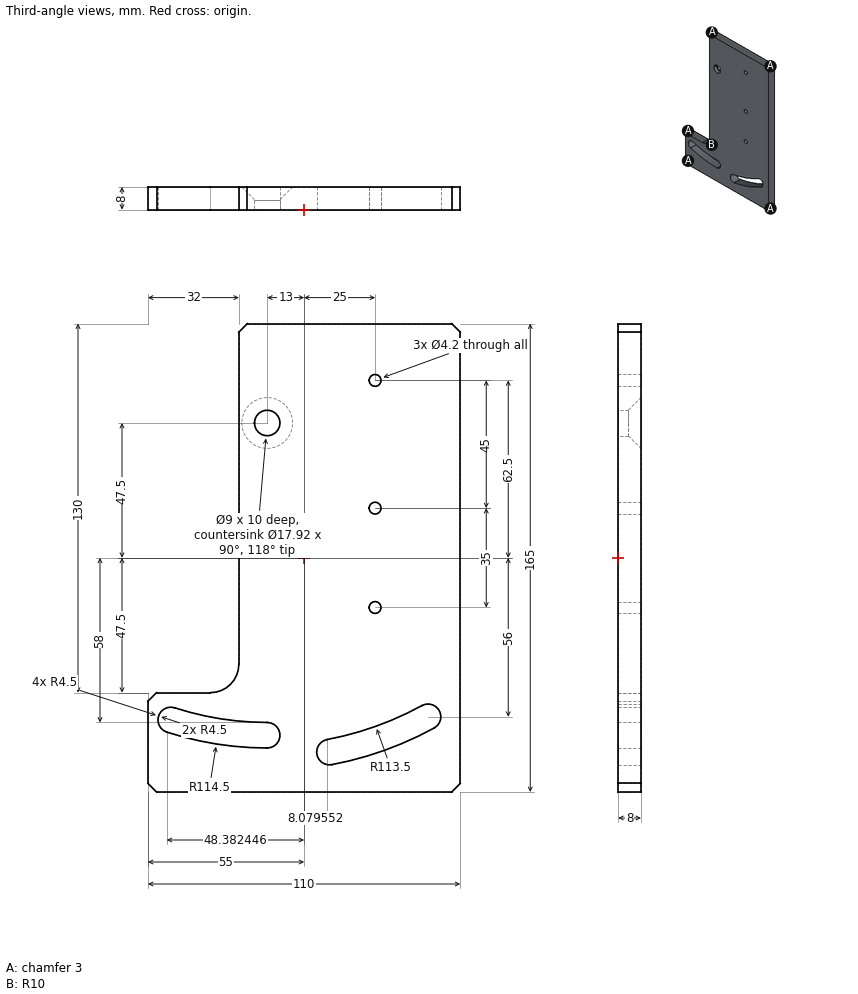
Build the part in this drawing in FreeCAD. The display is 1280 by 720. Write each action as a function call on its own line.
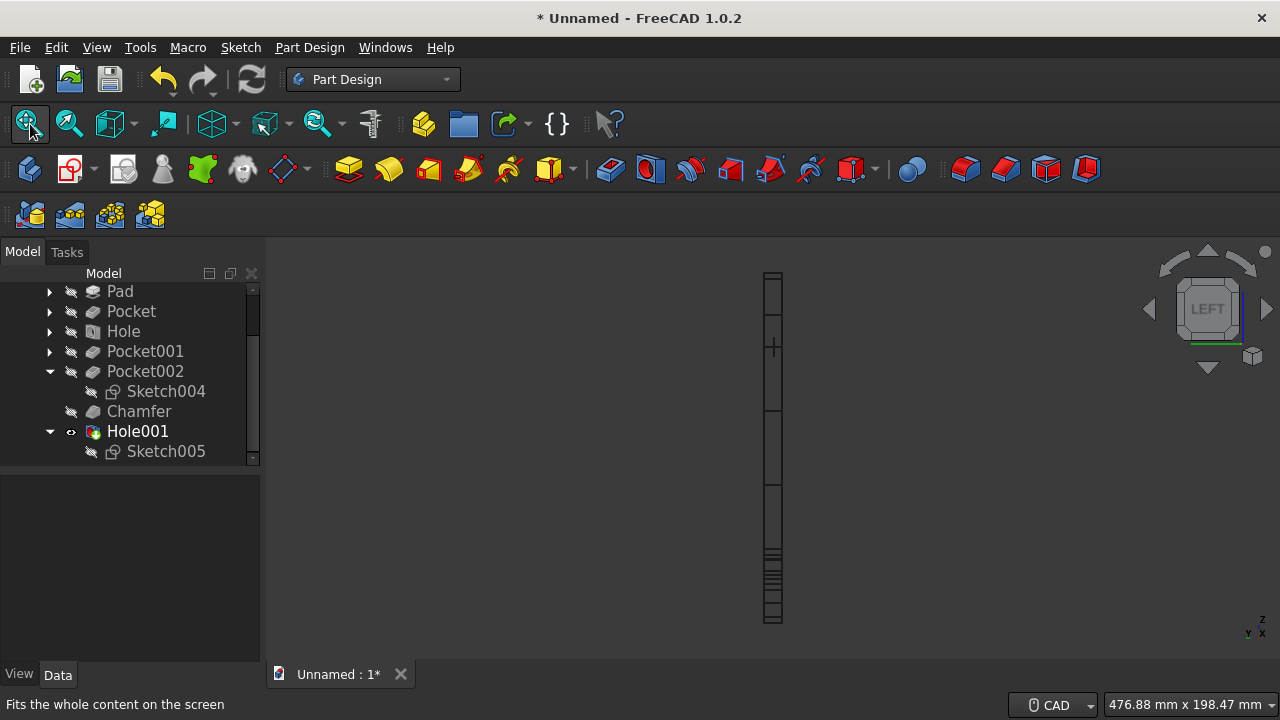
key(0)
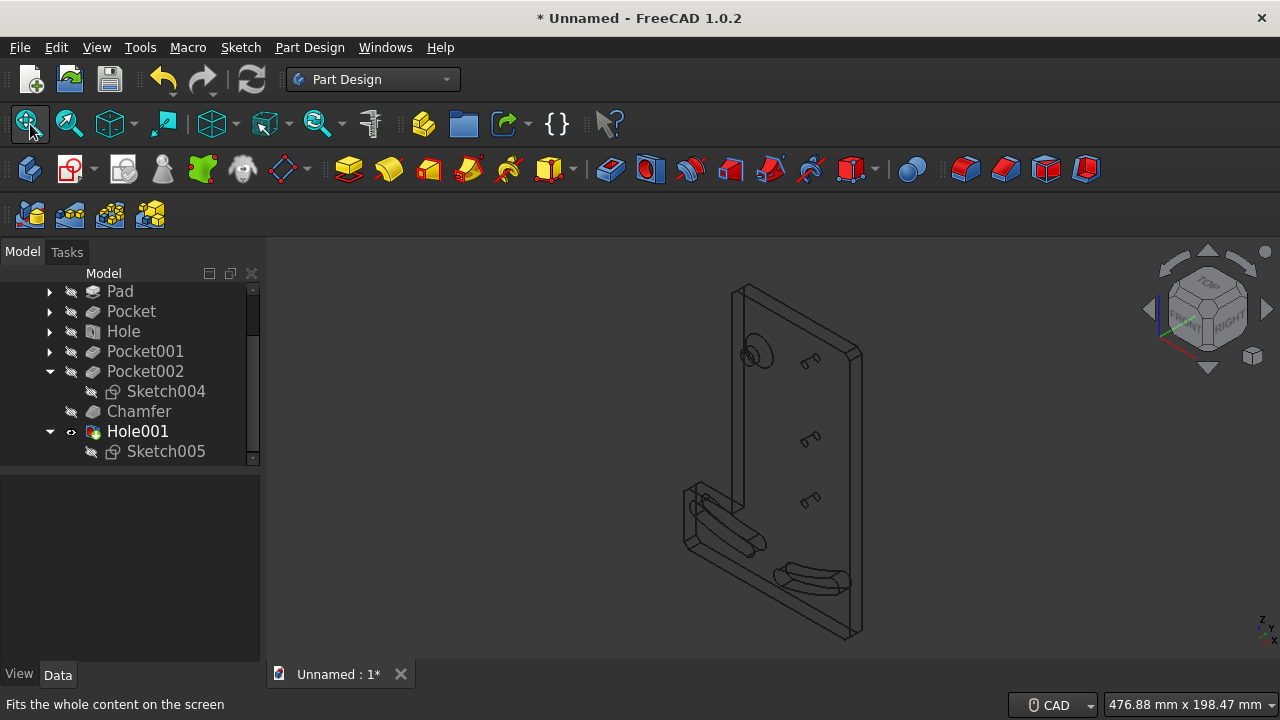
click(740, 509)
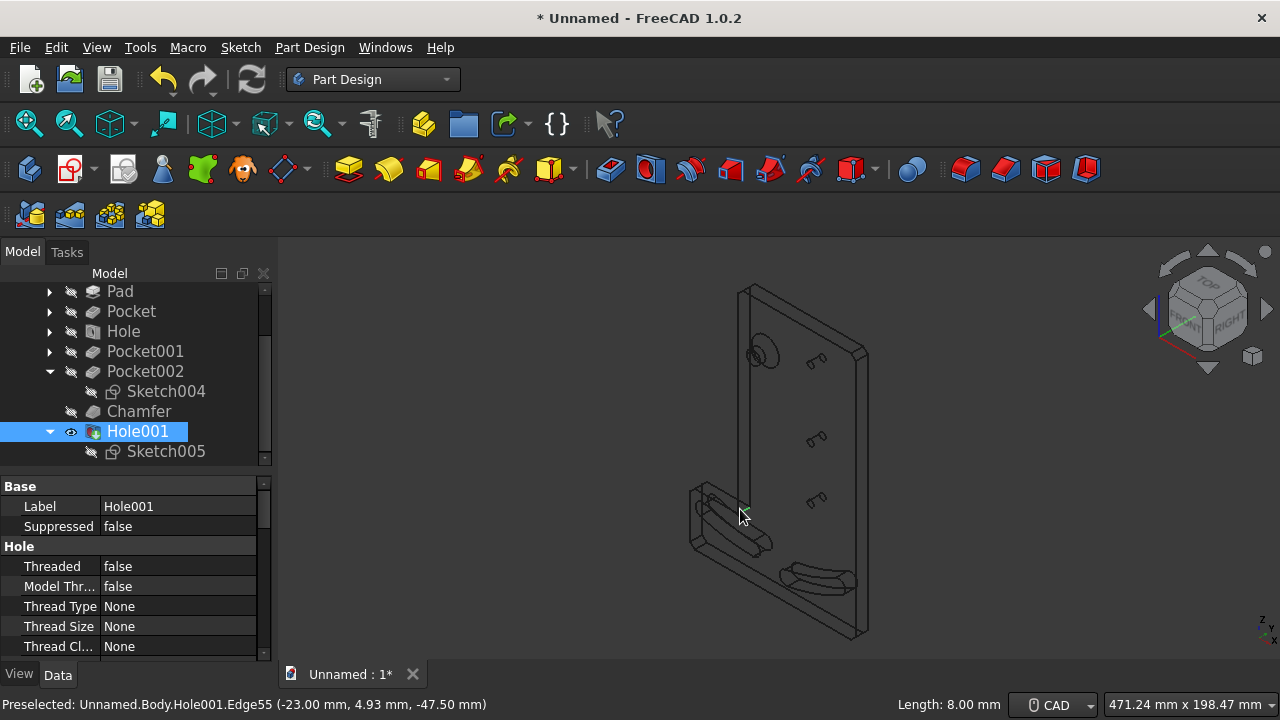
key(v)
key(1)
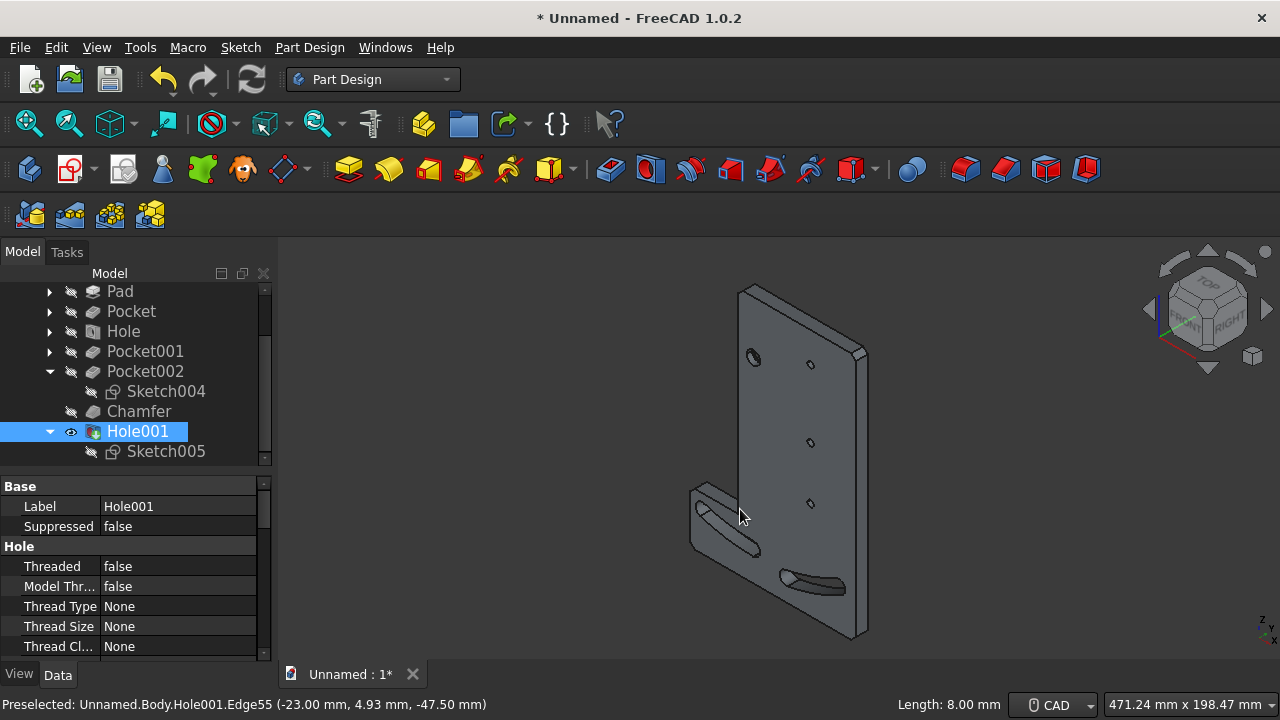
click(966, 170)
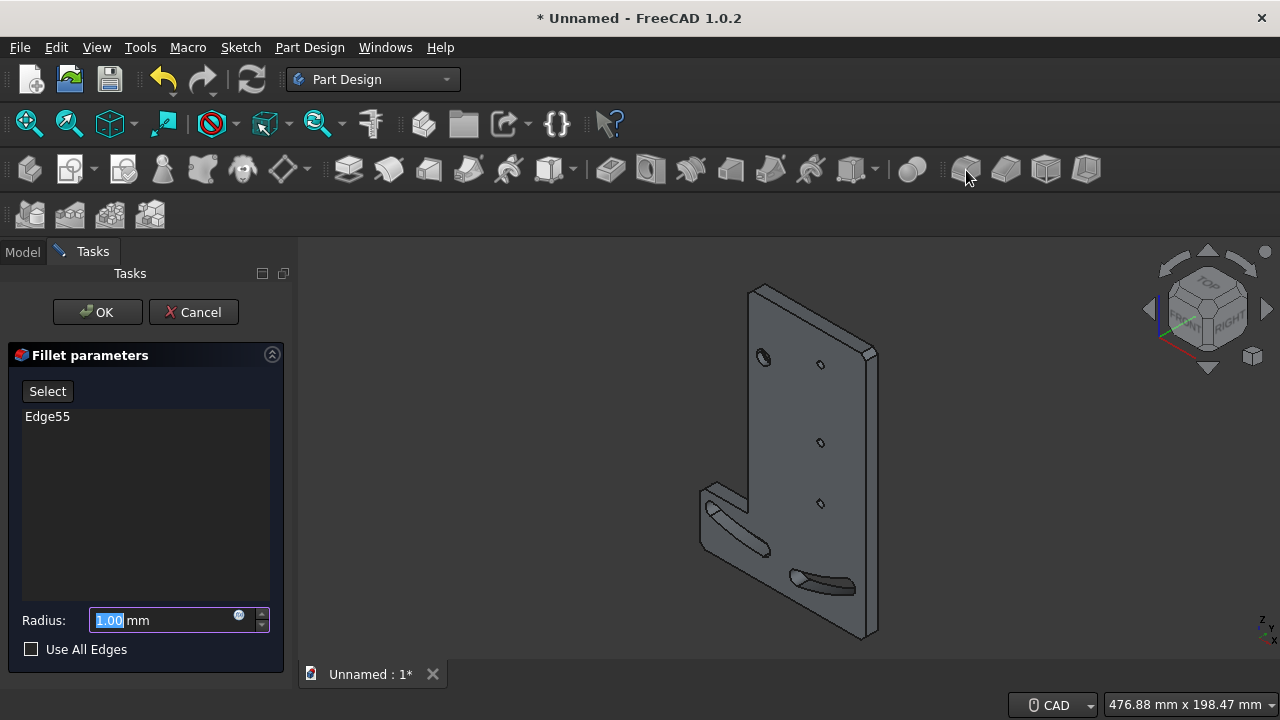
text(10)
key(Tab)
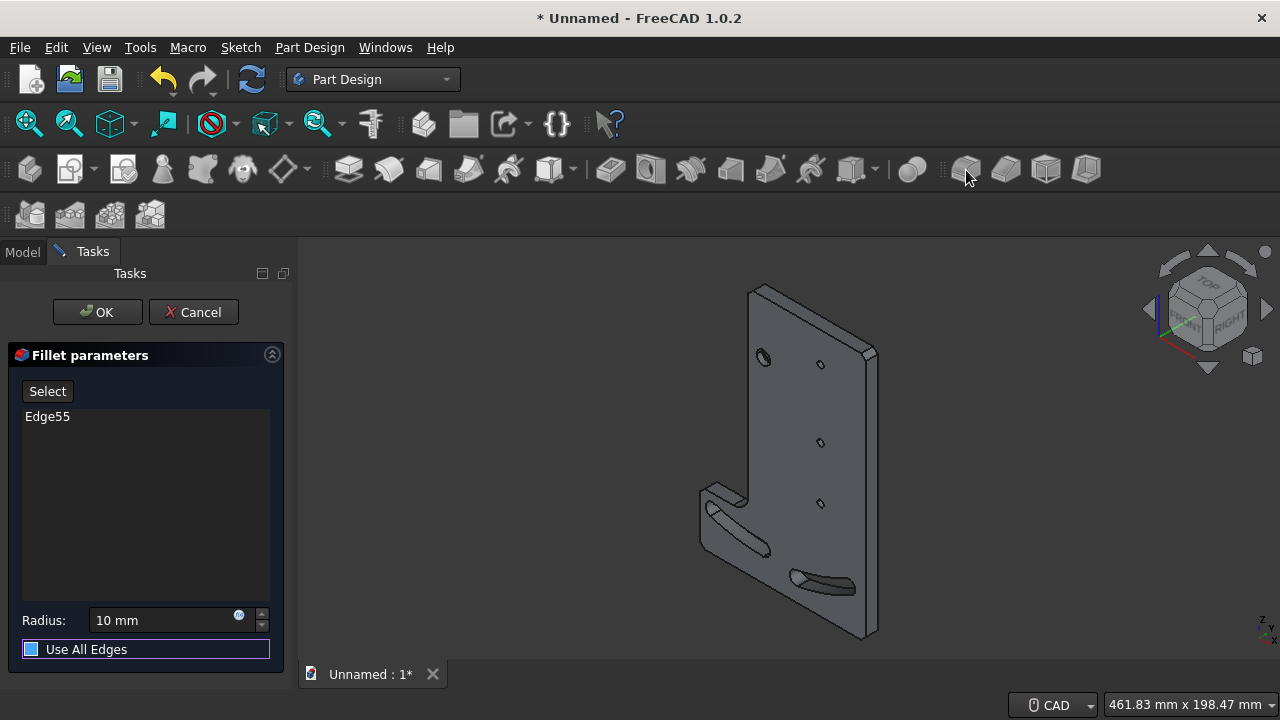
click(98, 312)